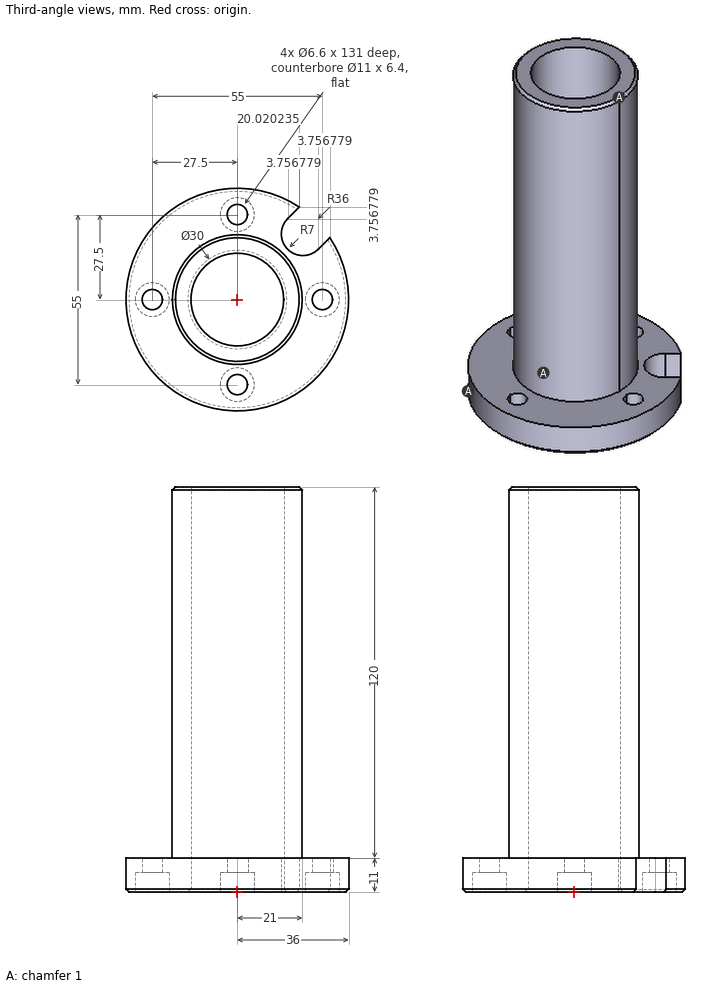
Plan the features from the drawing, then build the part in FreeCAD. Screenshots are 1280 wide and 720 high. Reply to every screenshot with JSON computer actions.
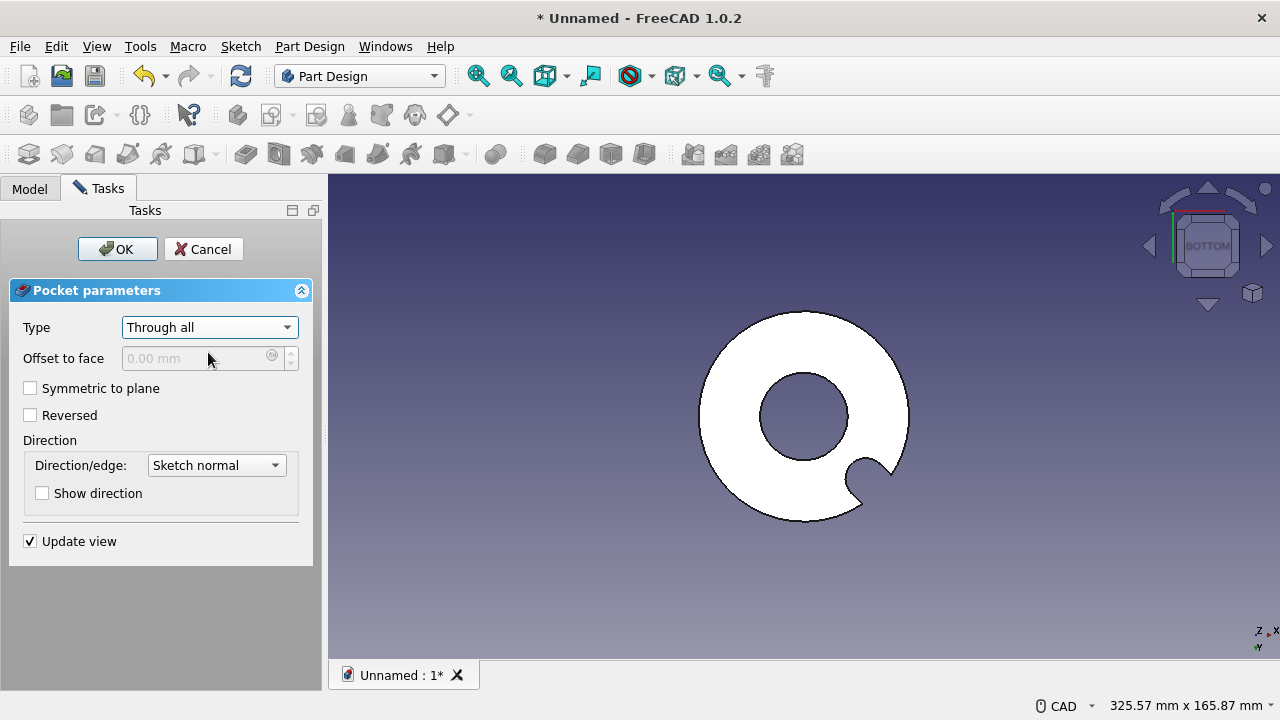
{"action": "left_click", "coordinate": [118, 249]}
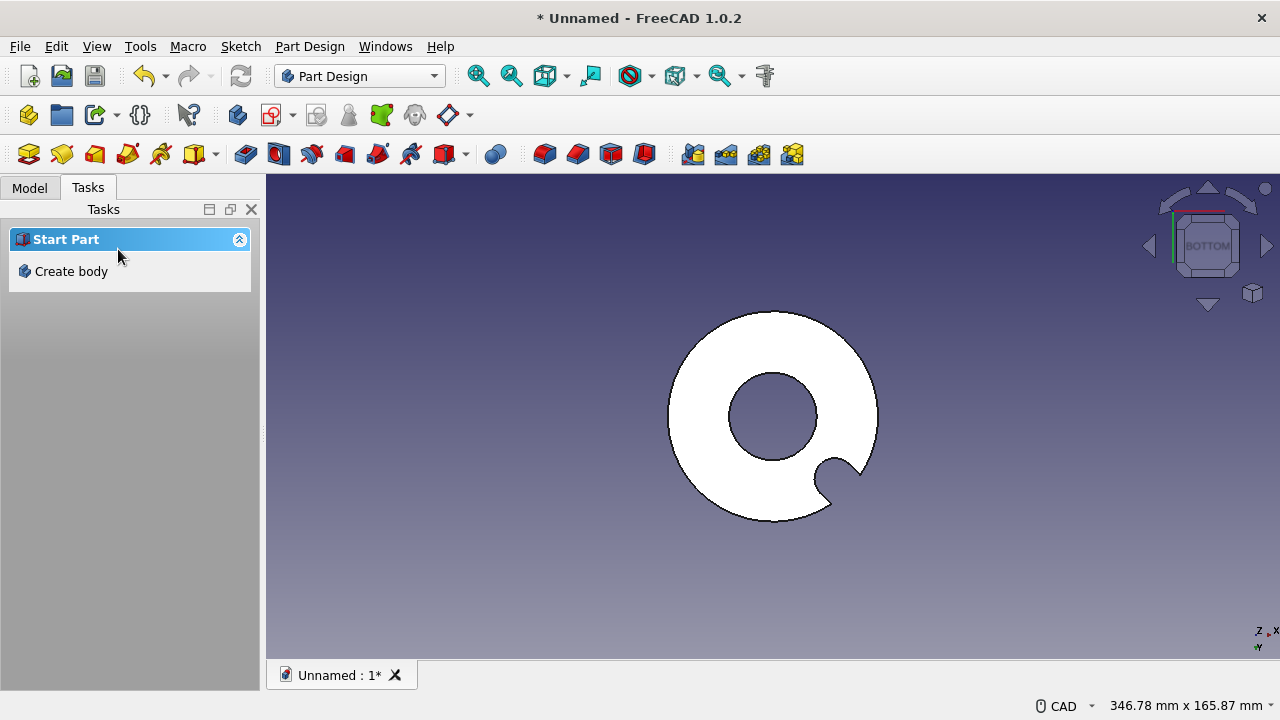
{"action": "left_click", "coordinate": [479, 76]}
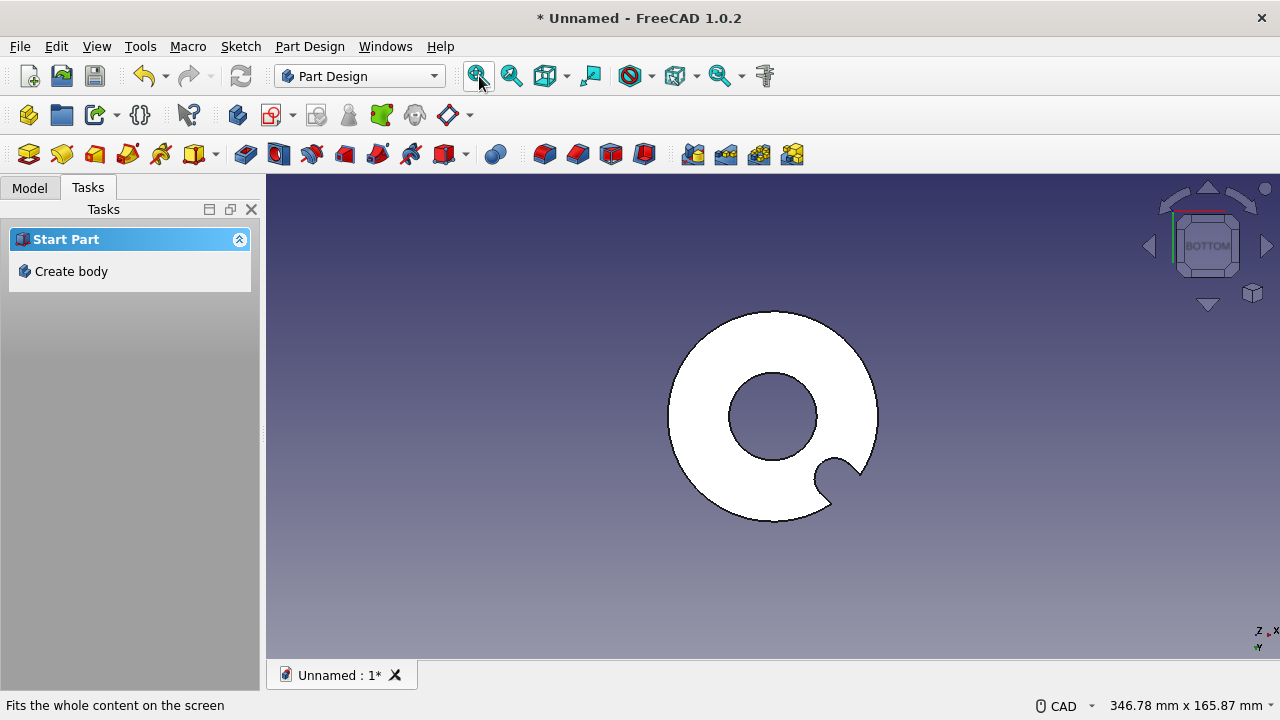
{"action": "left_click", "coordinate": [270, 116]}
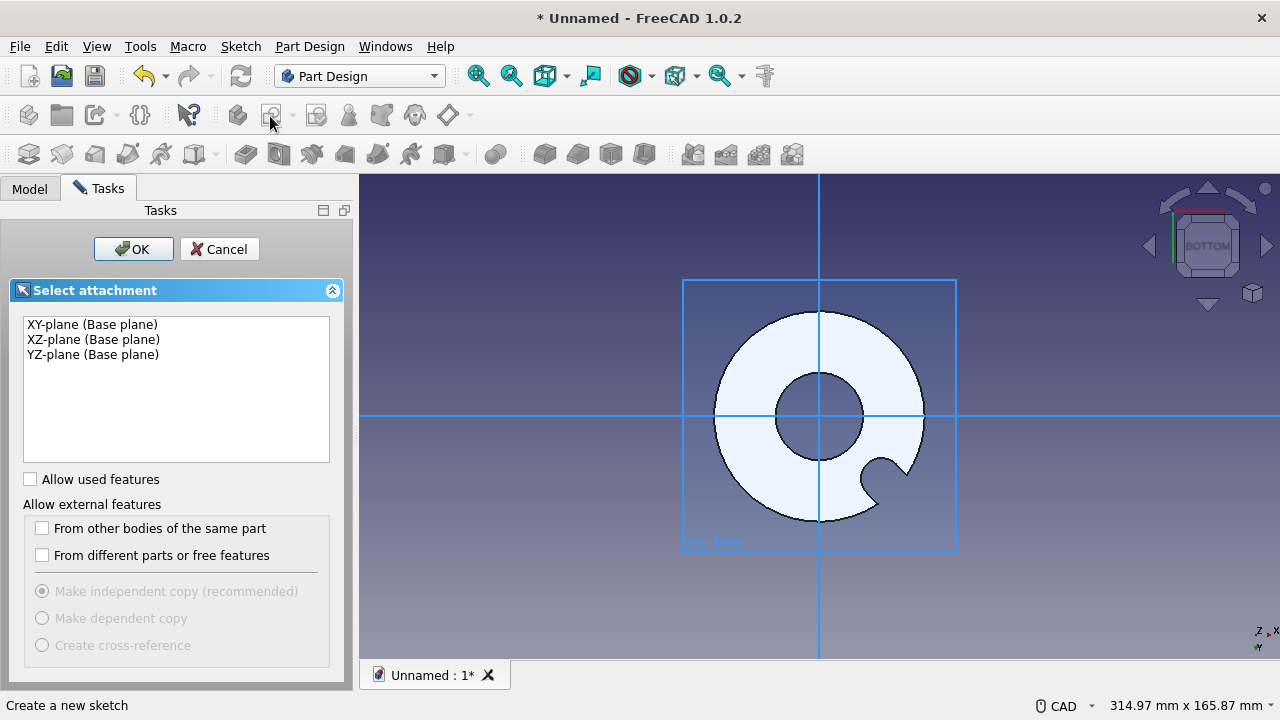
{"action": "left_click", "coordinate": [84, 324]}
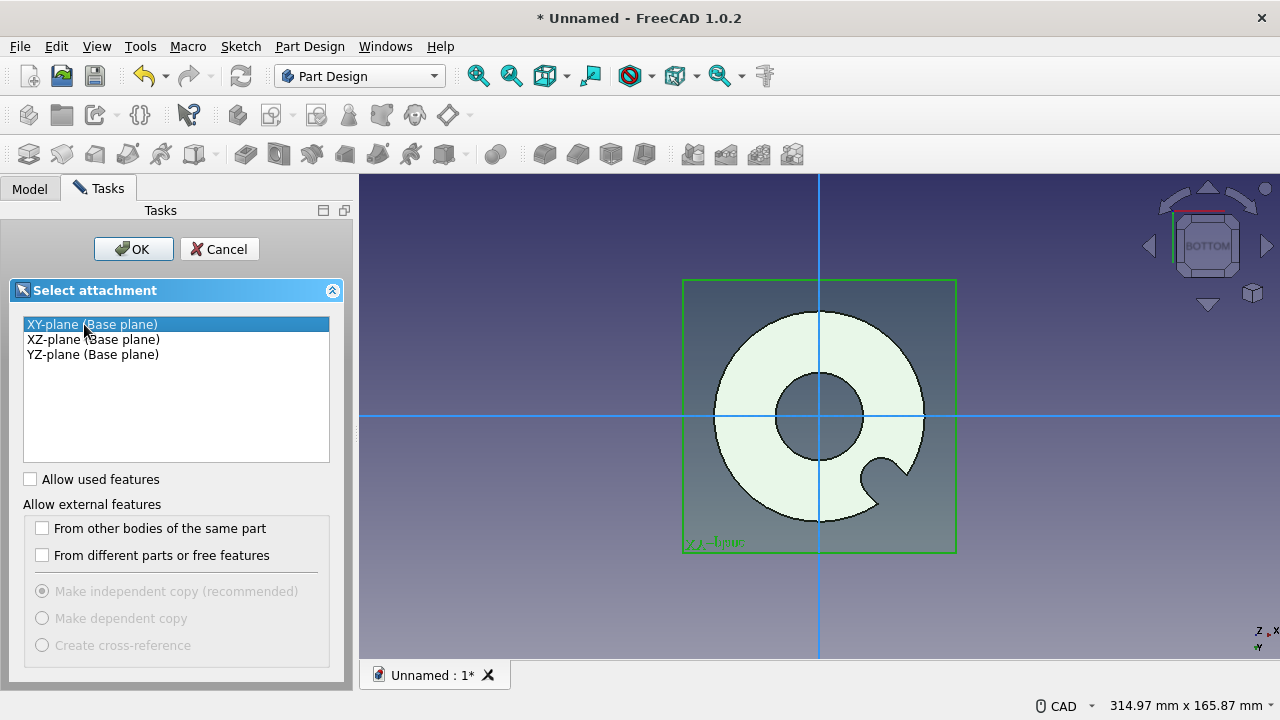
{"action": "left_click", "coordinate": [134, 249]}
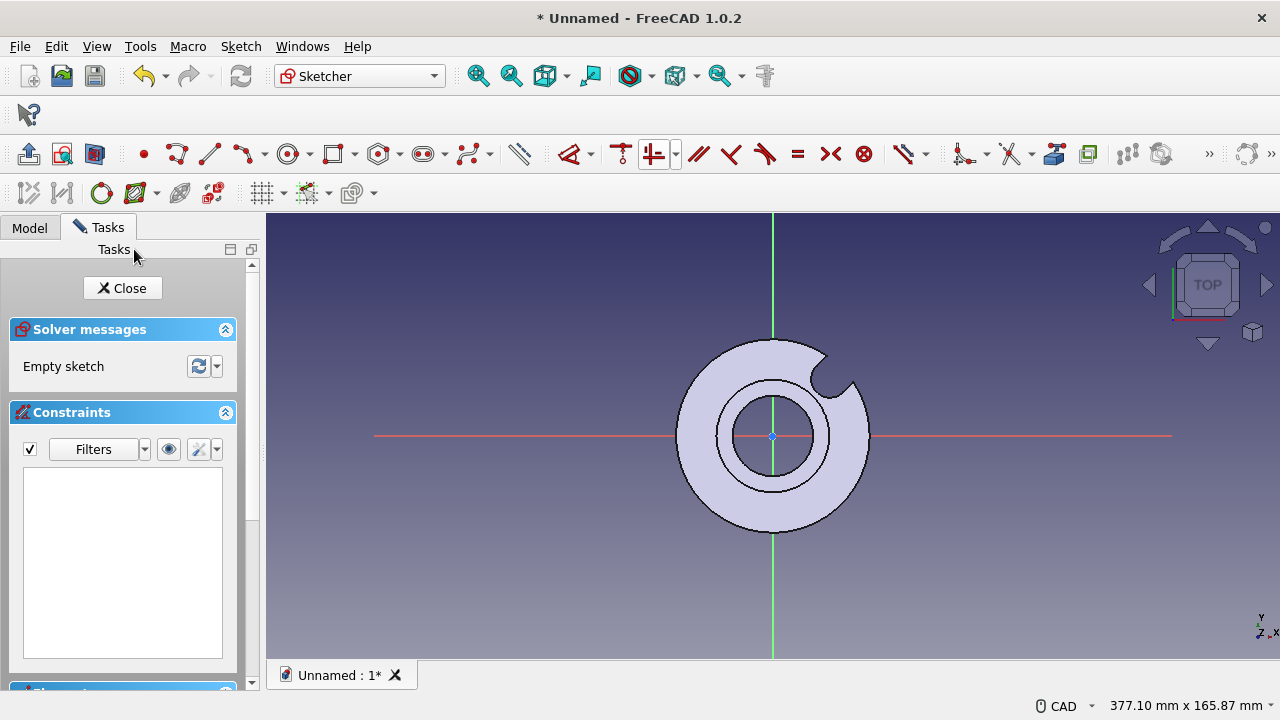
{"action": "key", "text": "q s"}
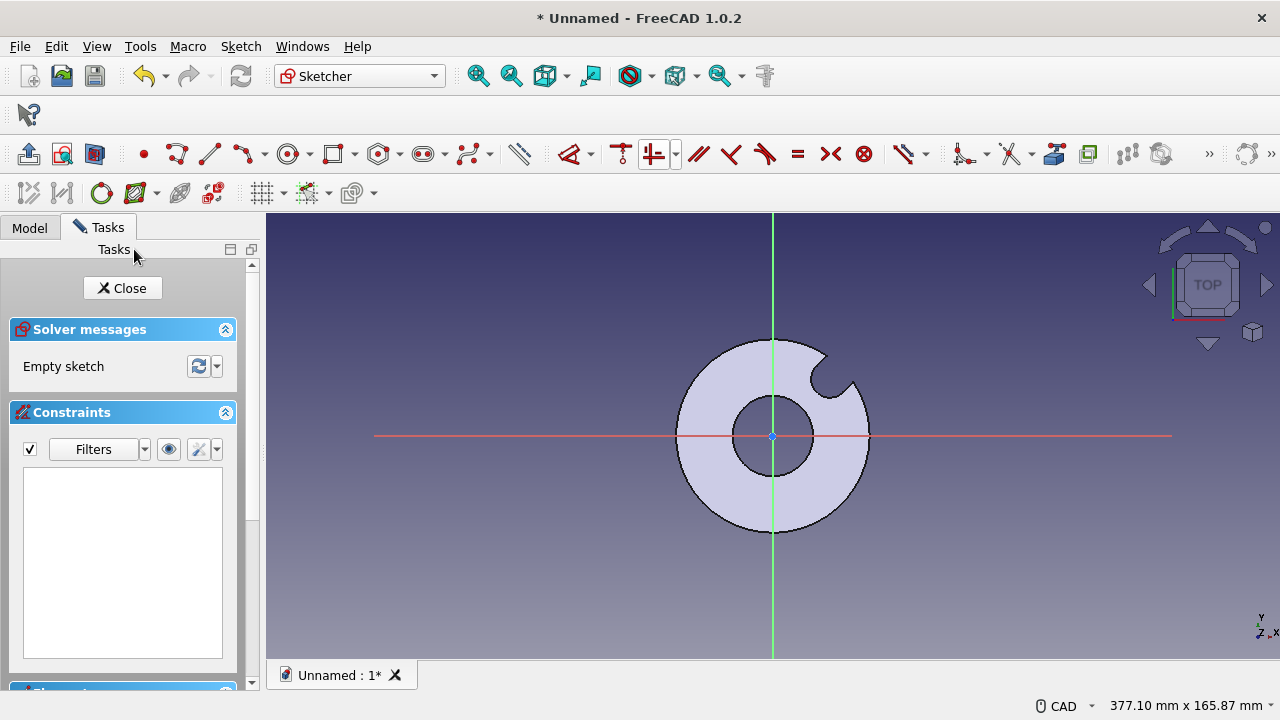
{"action": "scroll", "coordinate": [856, 436], "scroll_direction": "up", "scroll_amount": 3}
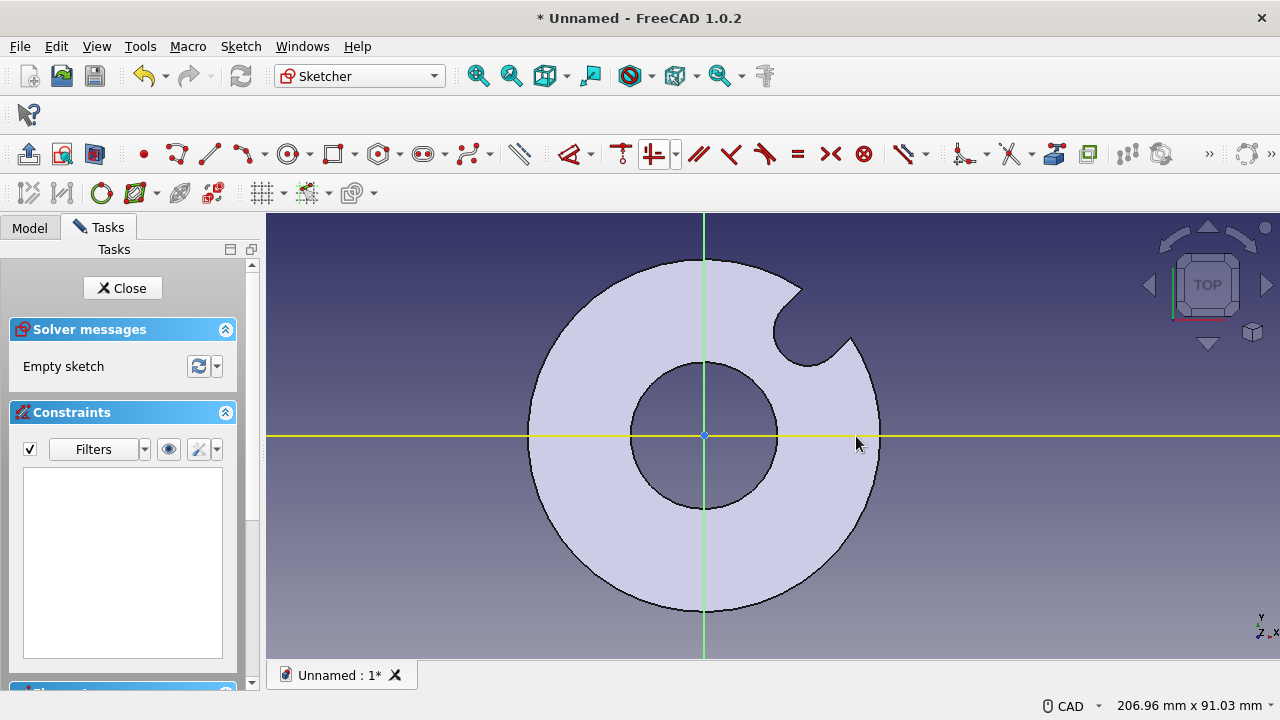
{"action": "left_click", "coordinate": [288, 154]}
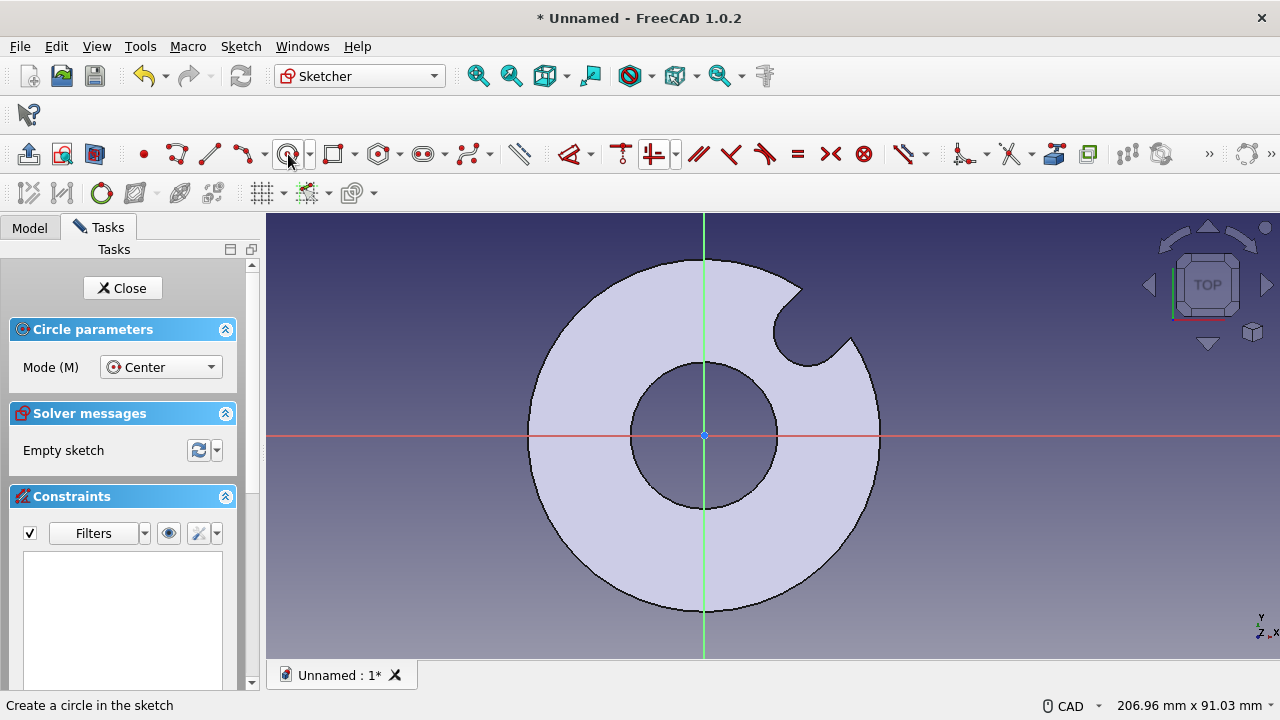
{"action": "scroll", "coordinate": [704, 301], "scroll_direction": "up", "scroll_amount": 2}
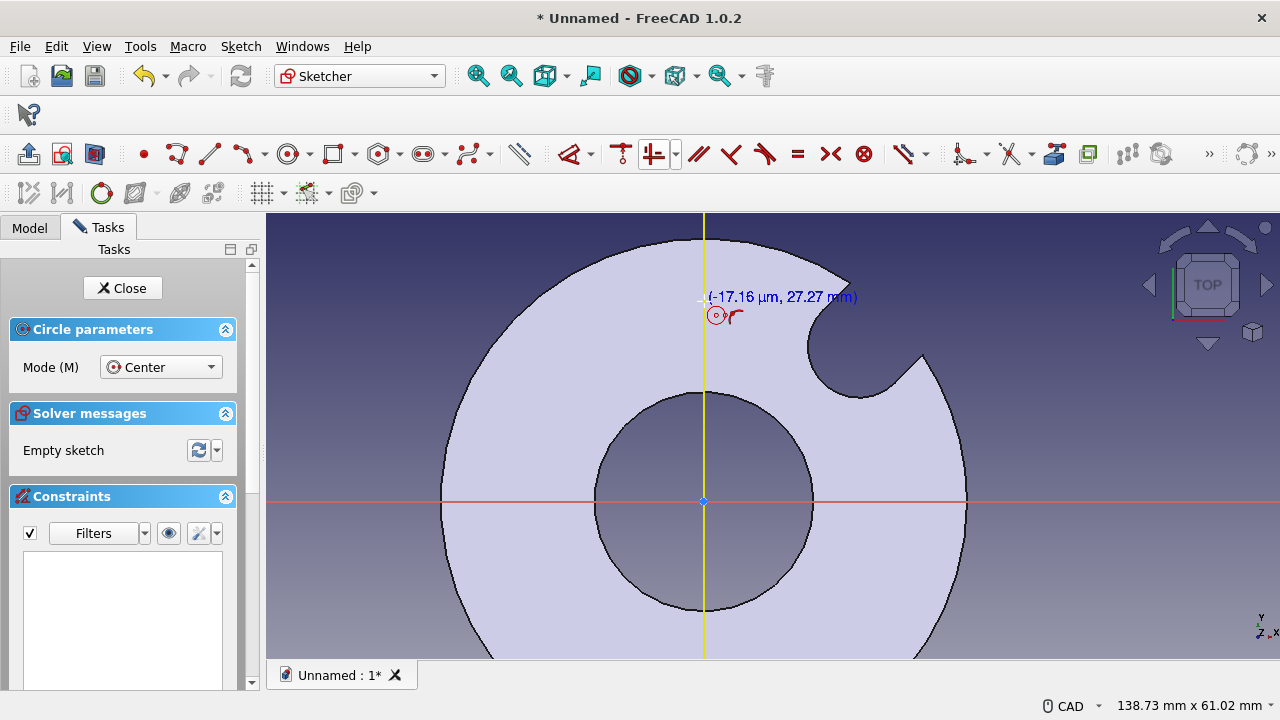
{"action": "left_click", "coordinate": [704, 301]}
{"action": "mouse_move", "coordinate": [721, 284]}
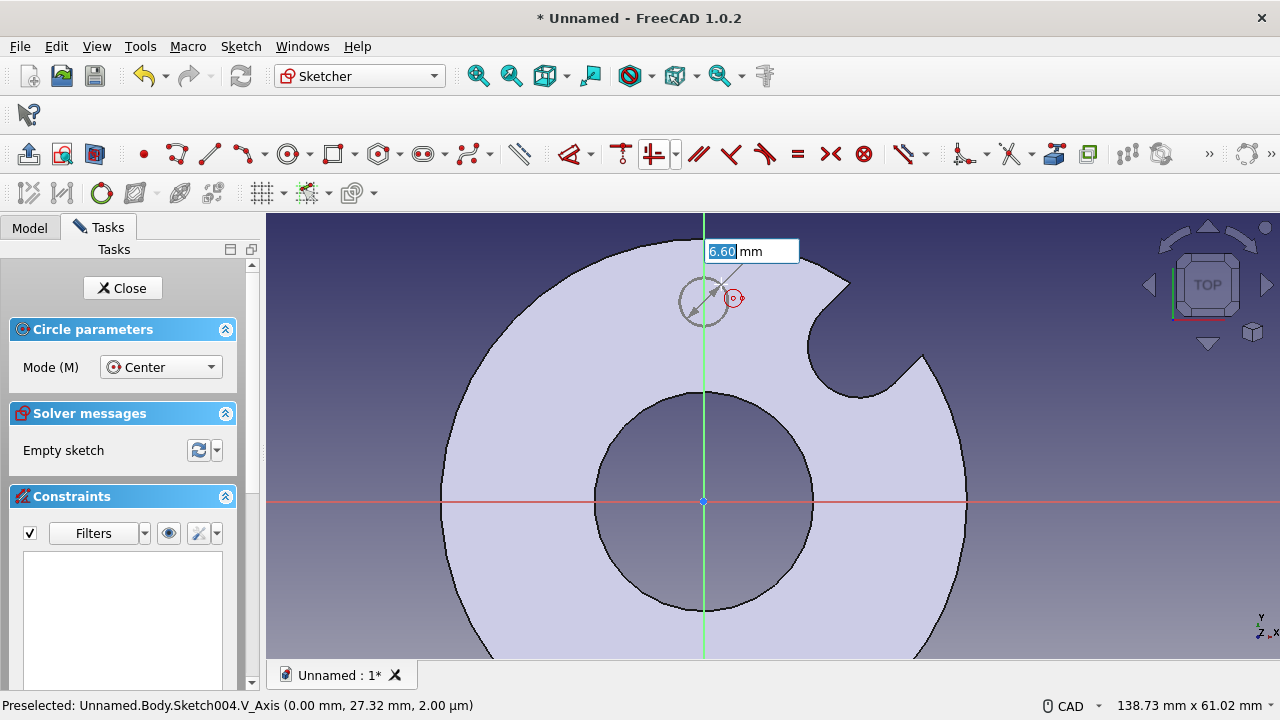
{"action": "type", "text": "6.6"}
{"action": "key", "text": "Return"}